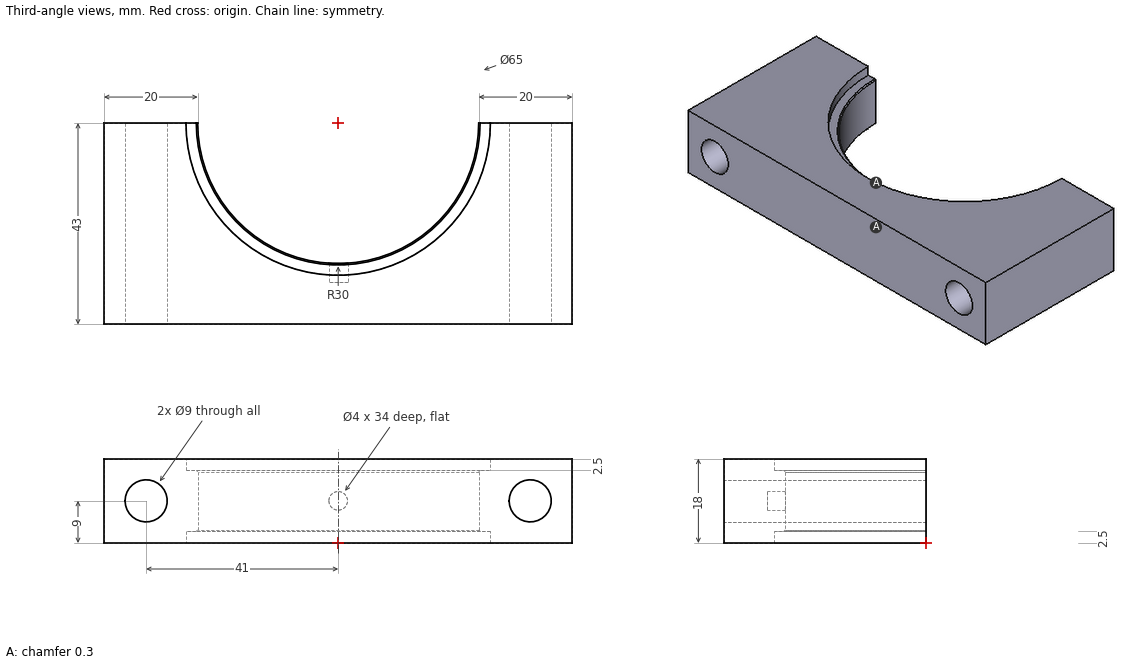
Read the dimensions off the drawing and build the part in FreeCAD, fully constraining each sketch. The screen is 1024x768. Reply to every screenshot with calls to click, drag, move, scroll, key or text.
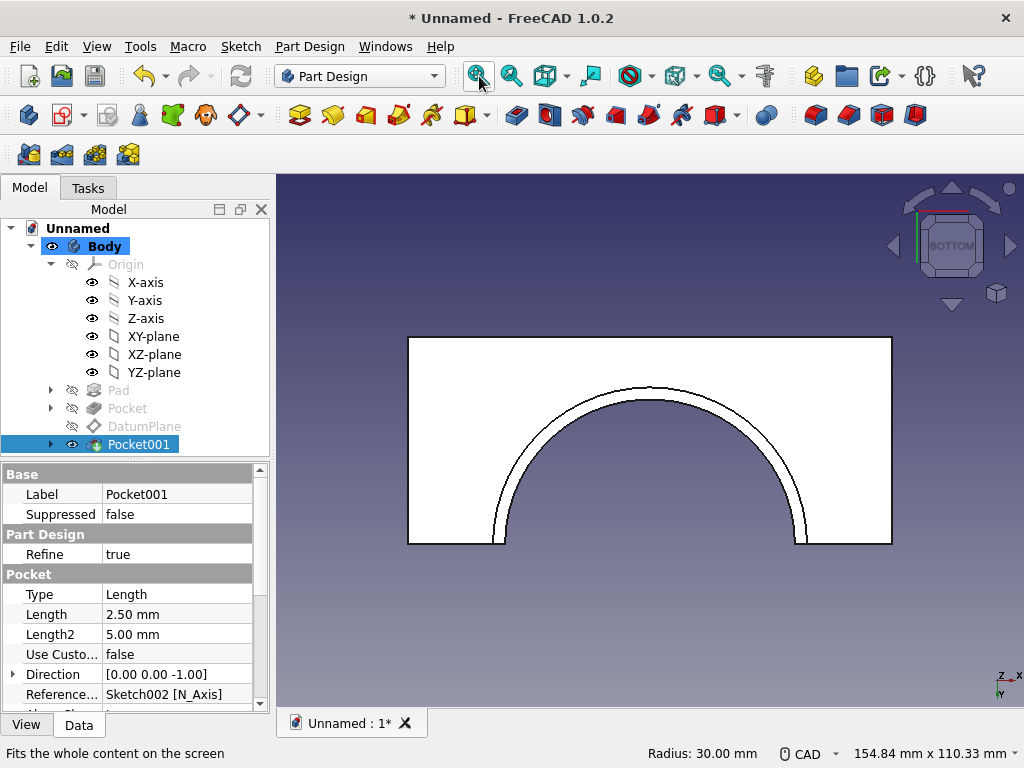
click(650, 398, ctrl)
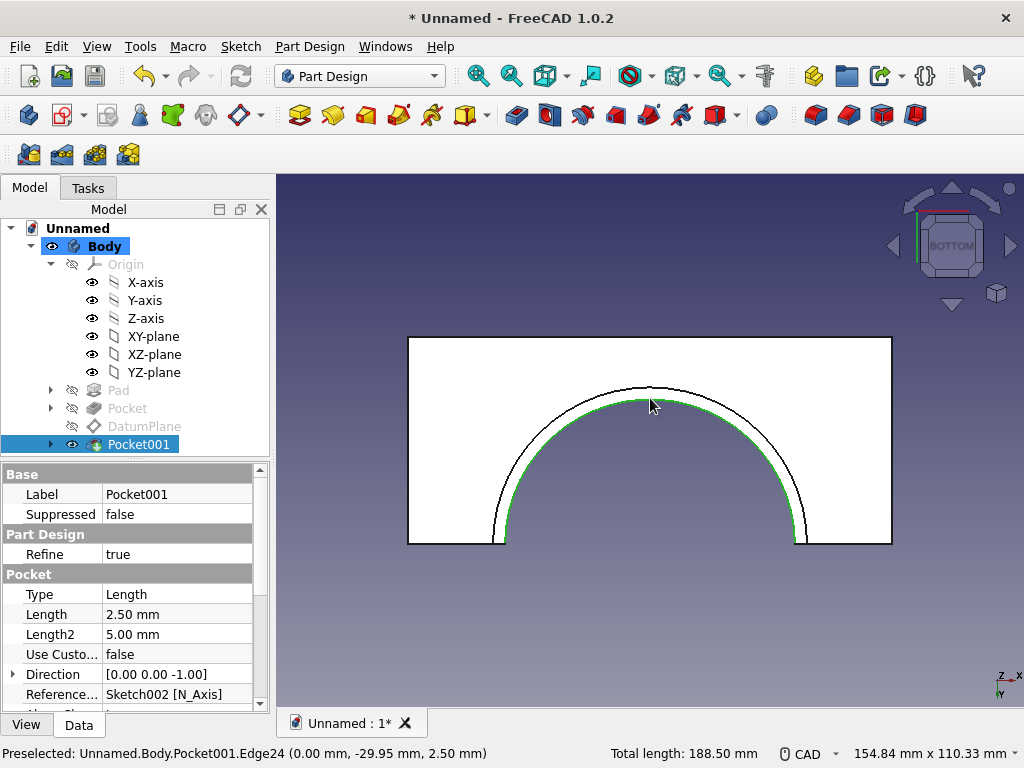
click(849, 116)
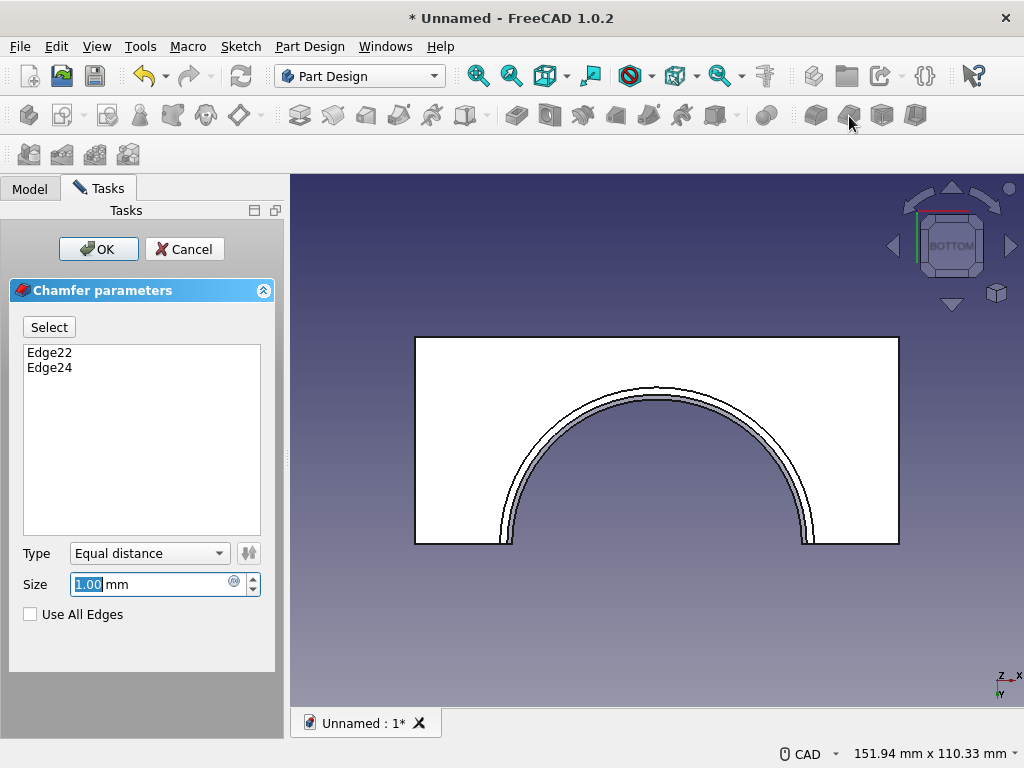
text(0.3)
key(Tab)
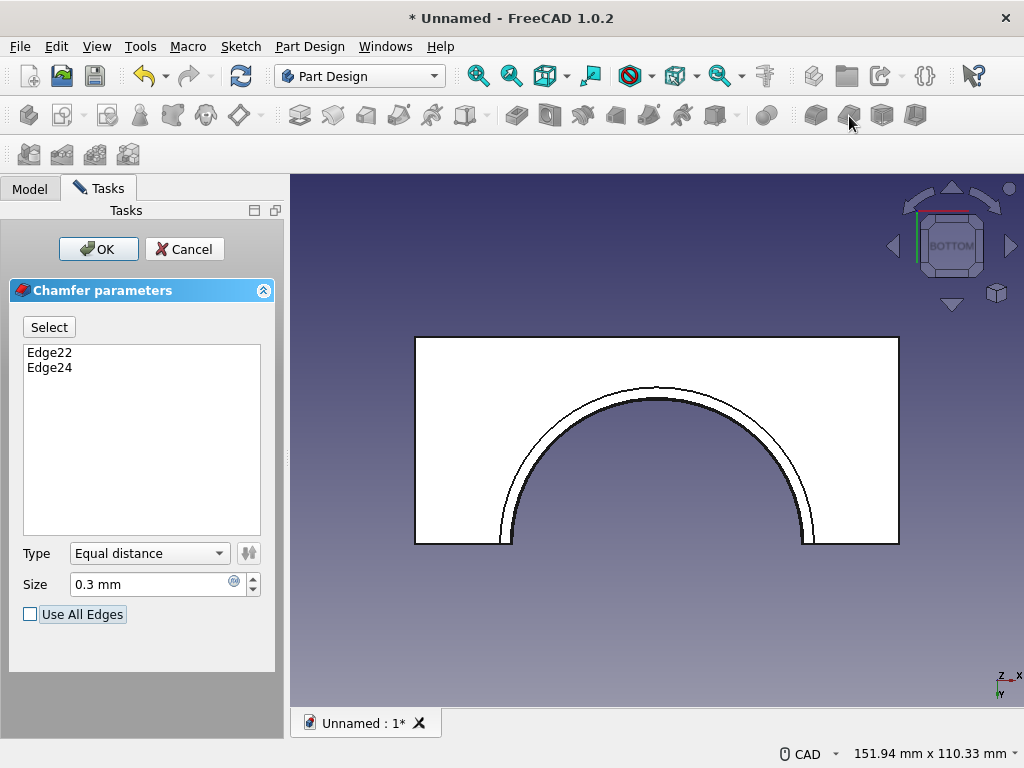
click(99, 249)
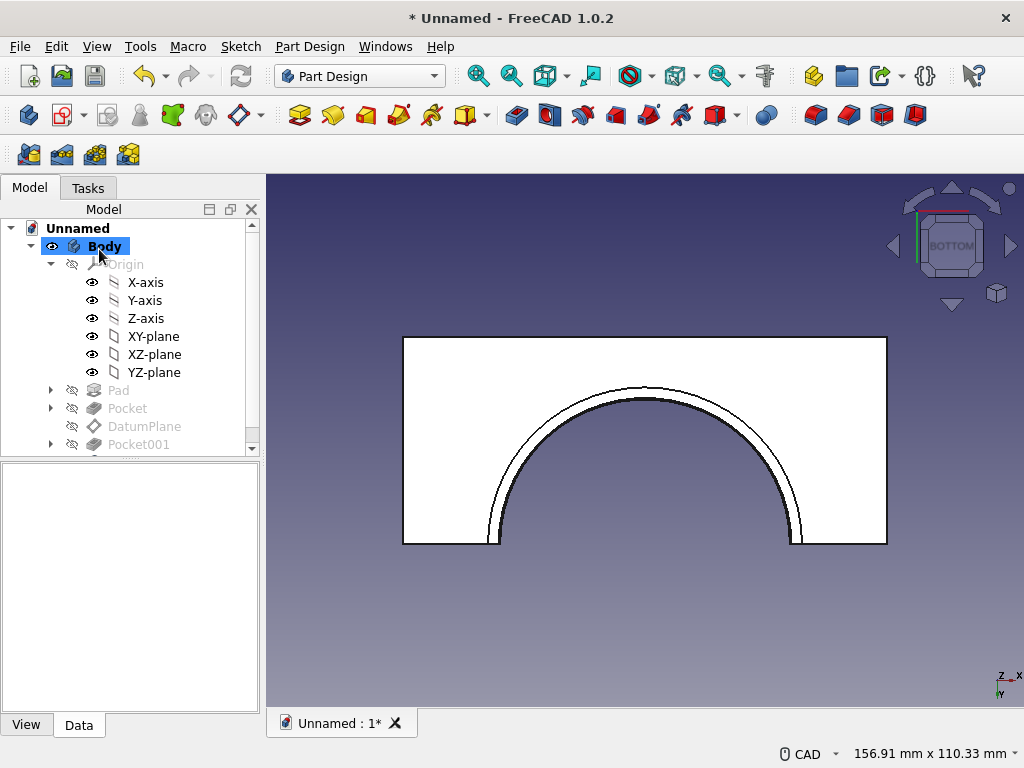
click(62, 116)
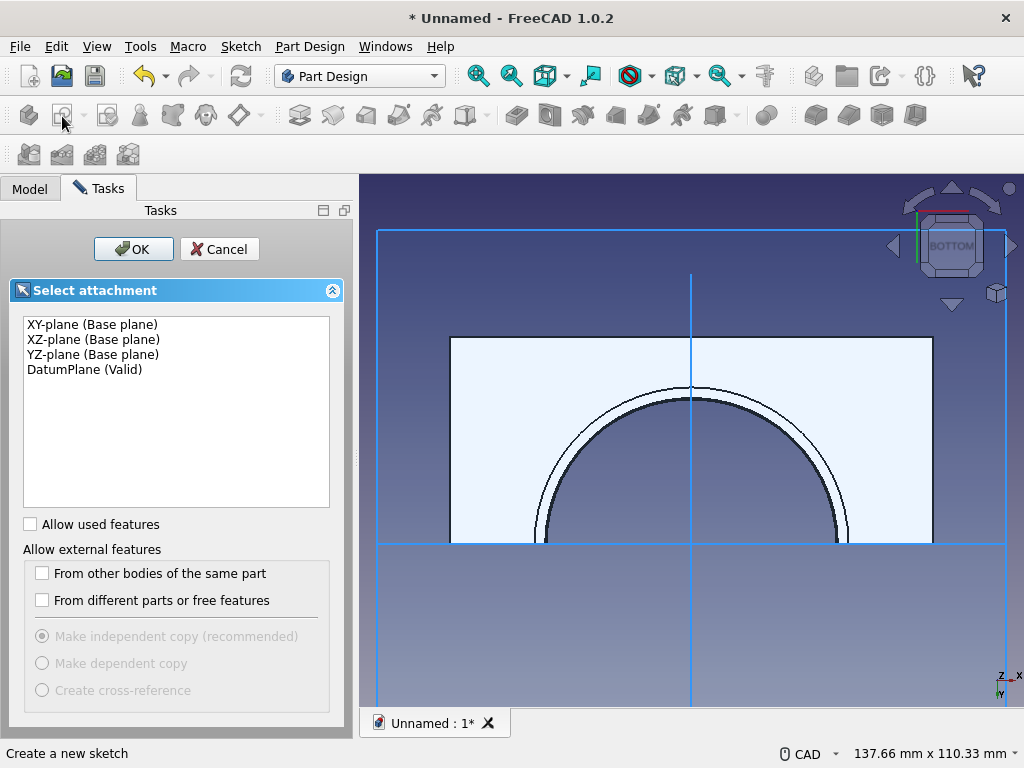
click(84, 340)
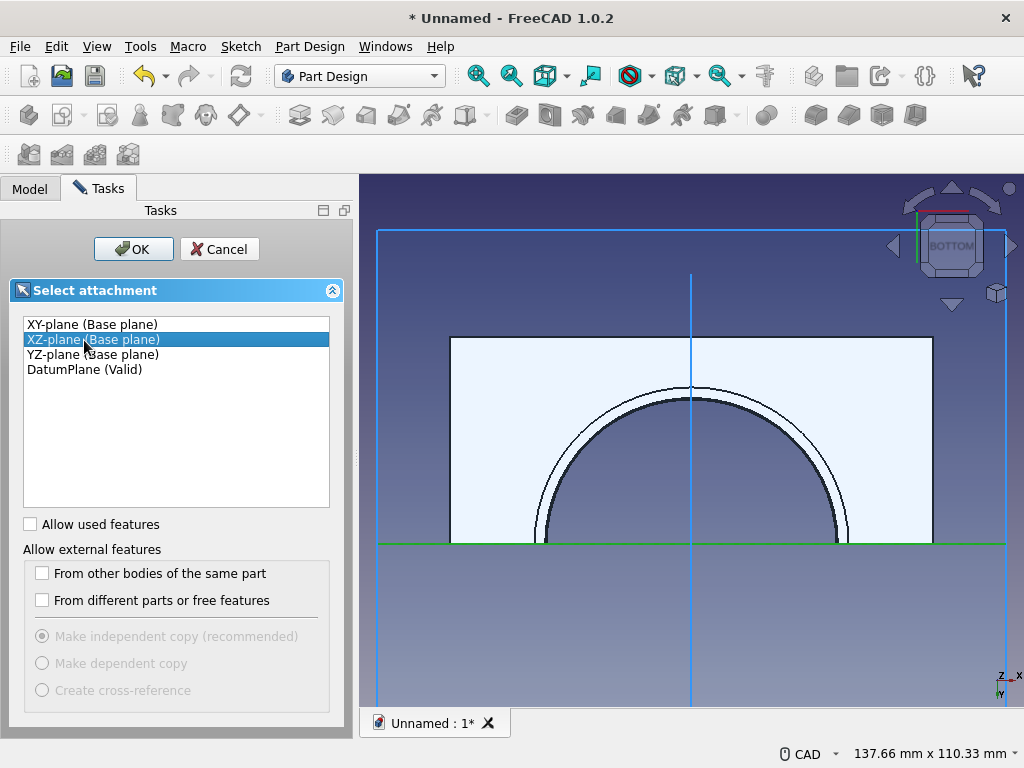
click(134, 249)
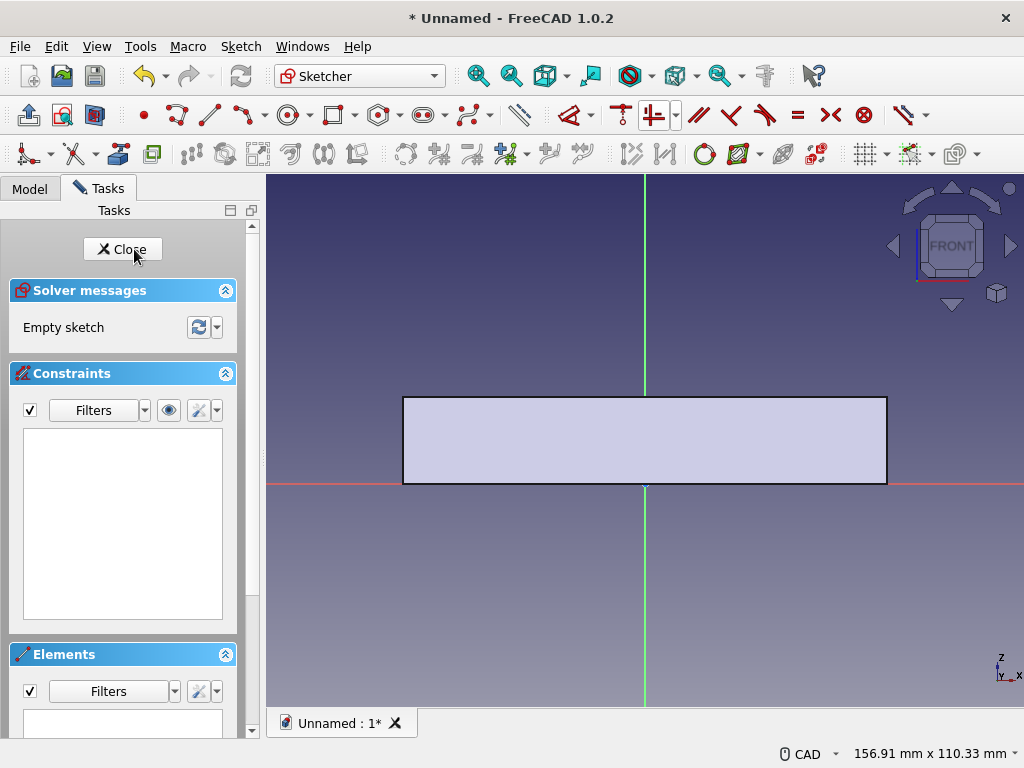
click(95, 116)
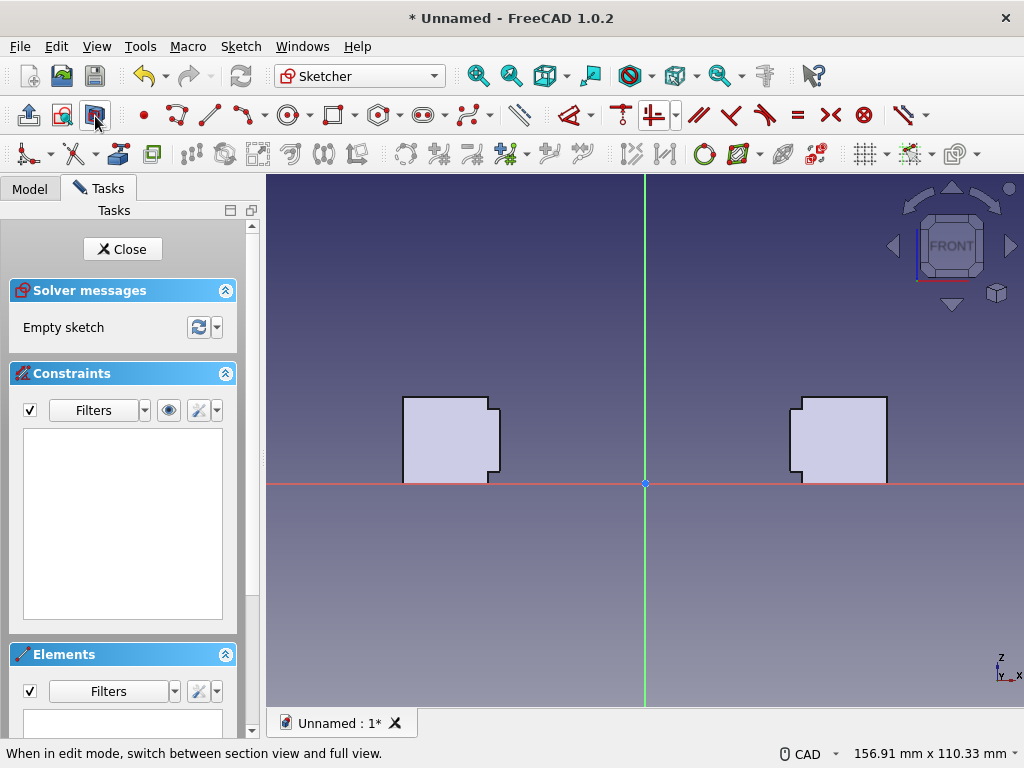
scroll(294, 391, down, 1)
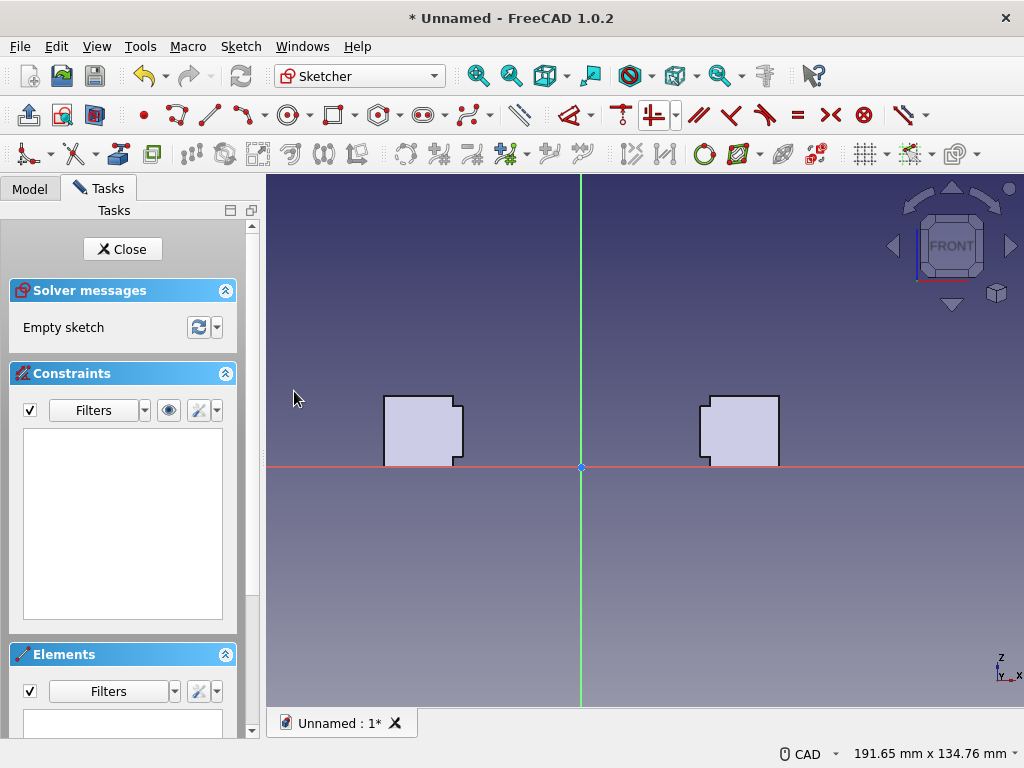
click(288, 116)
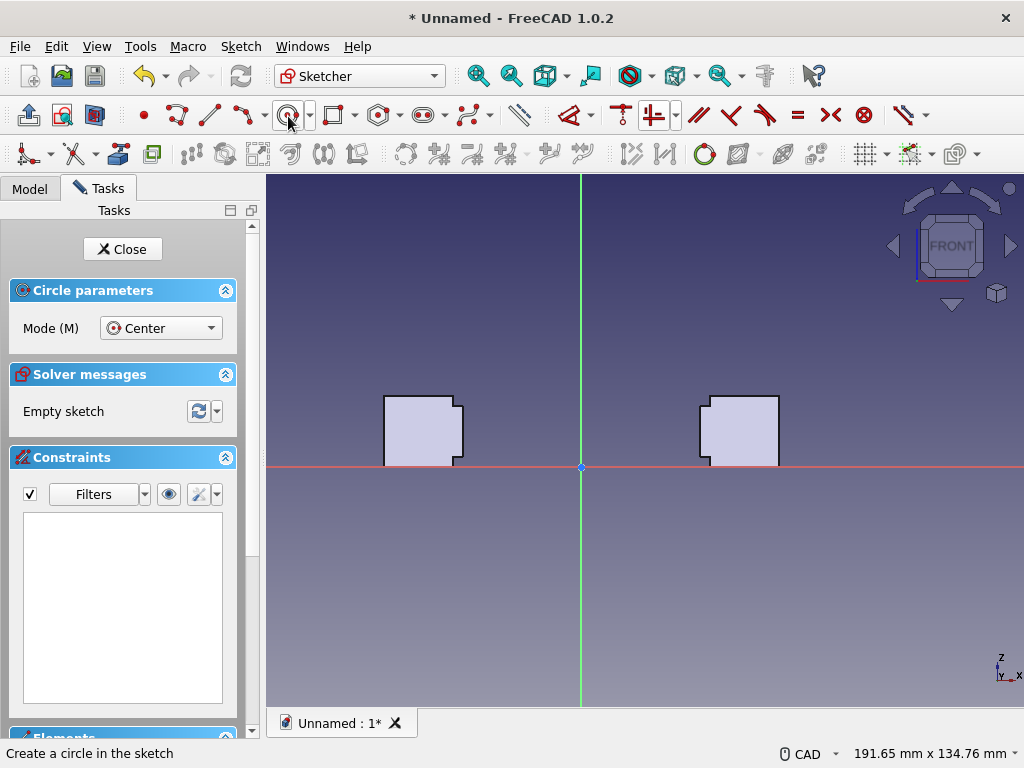
scroll(419, 432, up, 2)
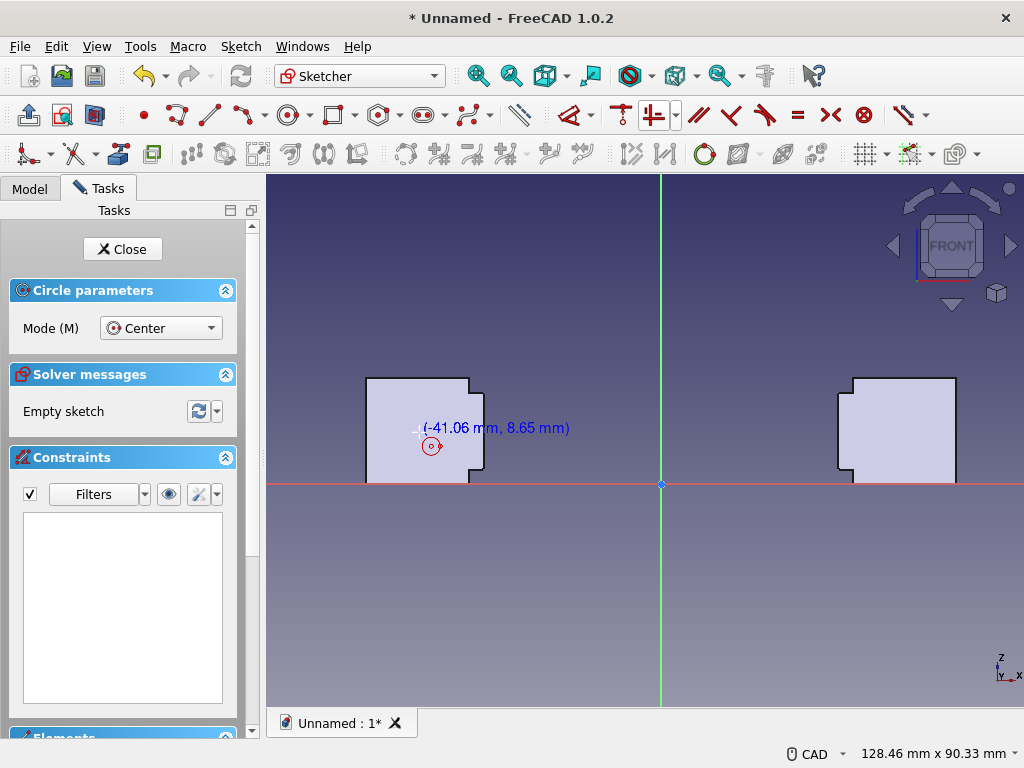
click(419, 431)
move(438, 412)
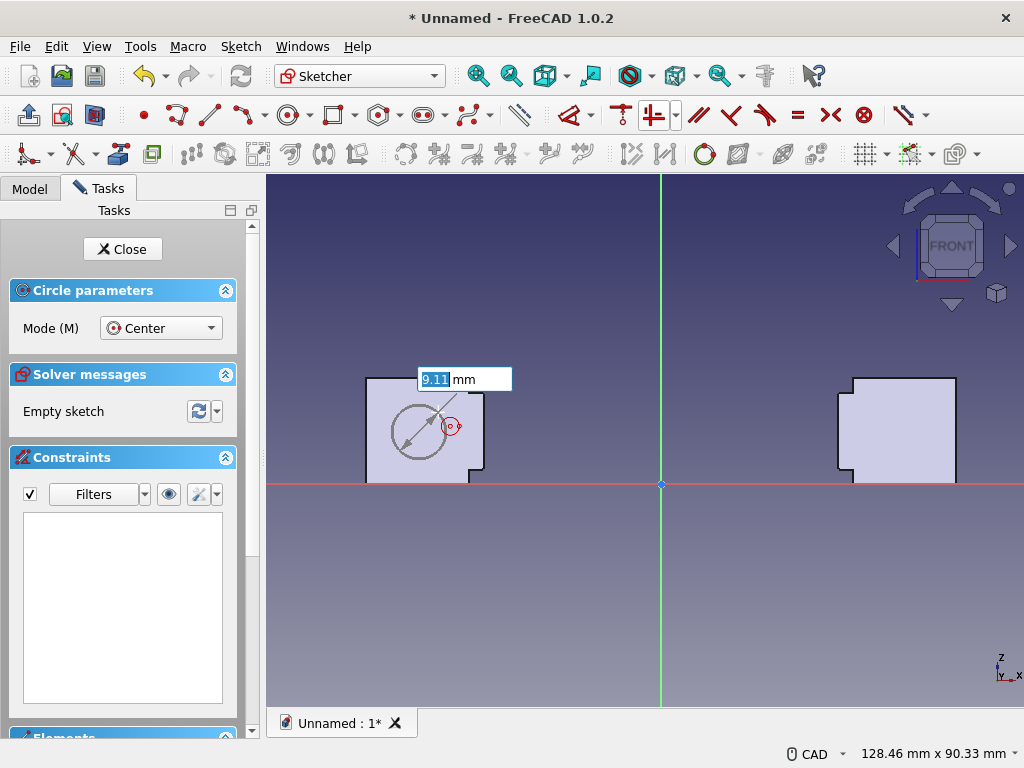
text(9)
key(Return)